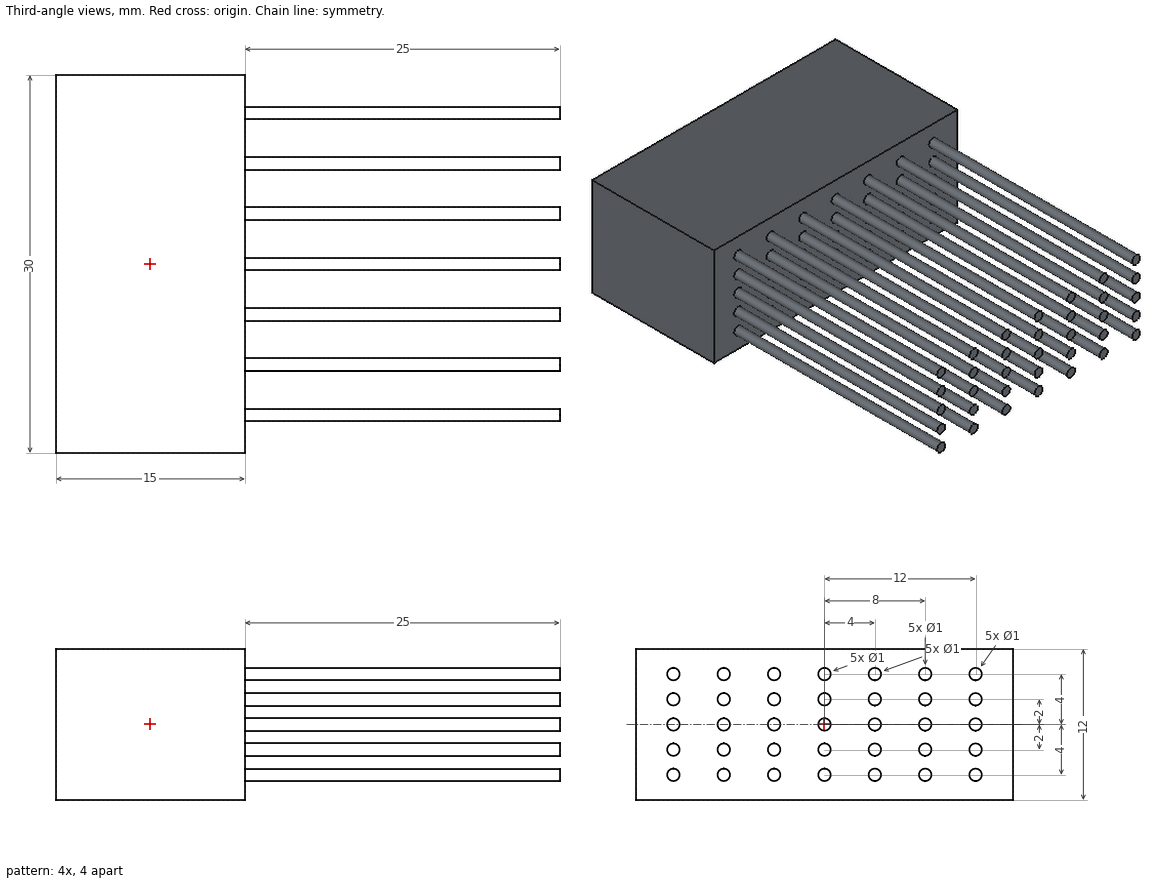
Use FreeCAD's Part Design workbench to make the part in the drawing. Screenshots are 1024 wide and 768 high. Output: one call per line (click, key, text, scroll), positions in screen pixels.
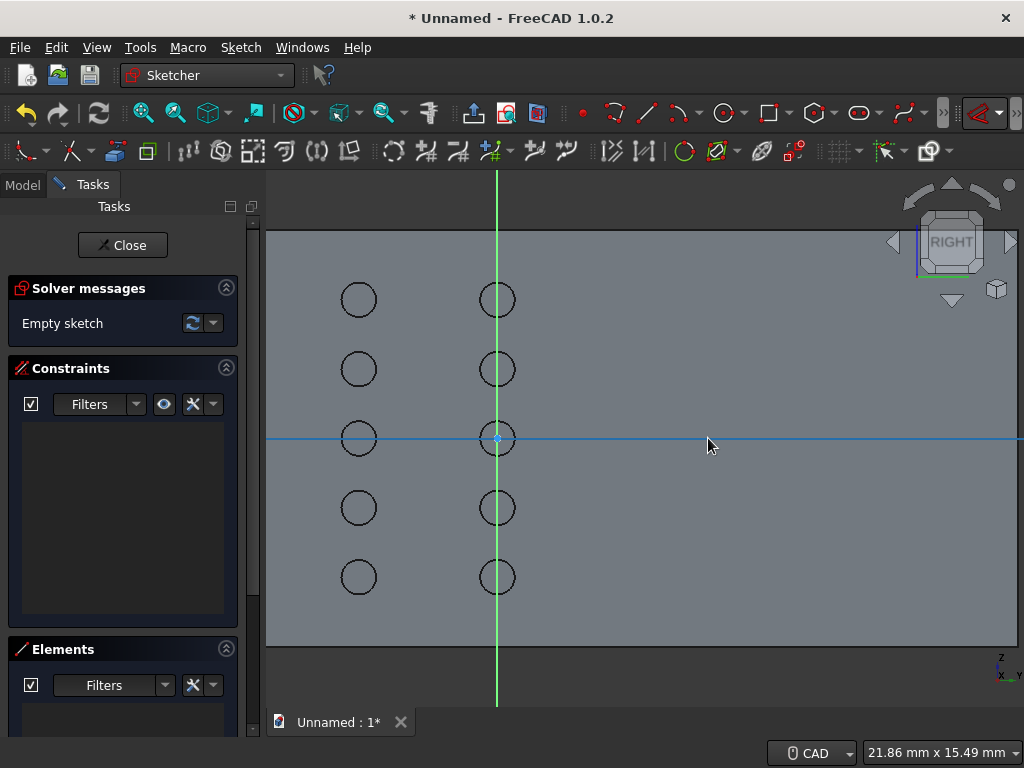
key(g)
key(c)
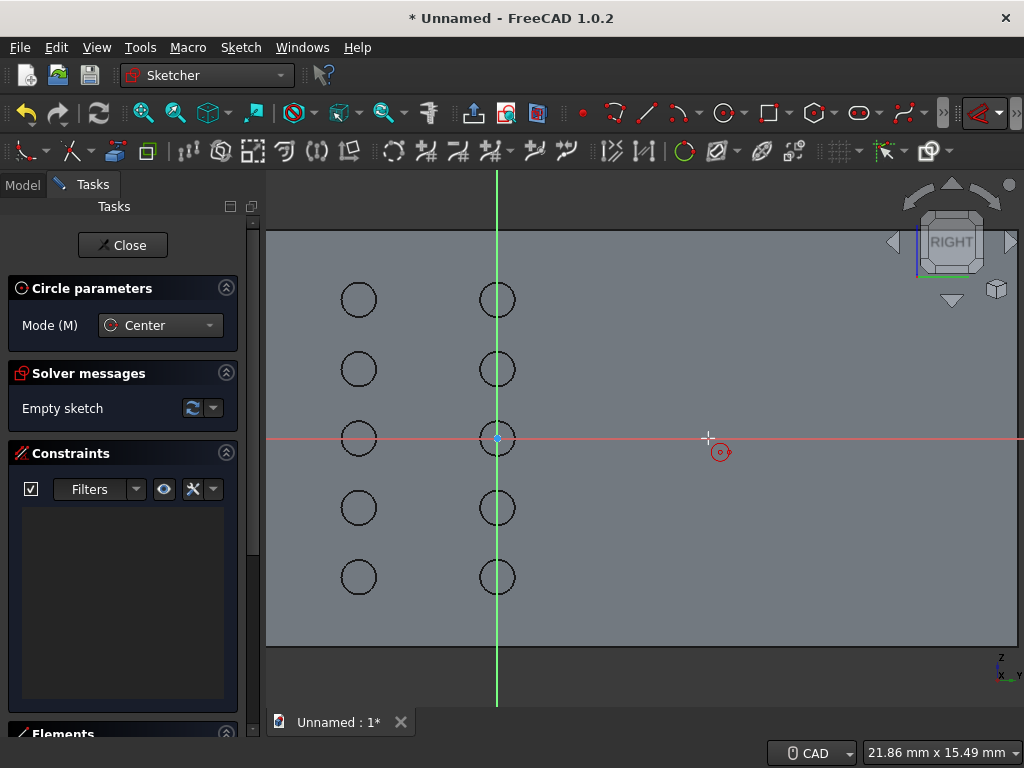
scroll(636, 300, up, 2)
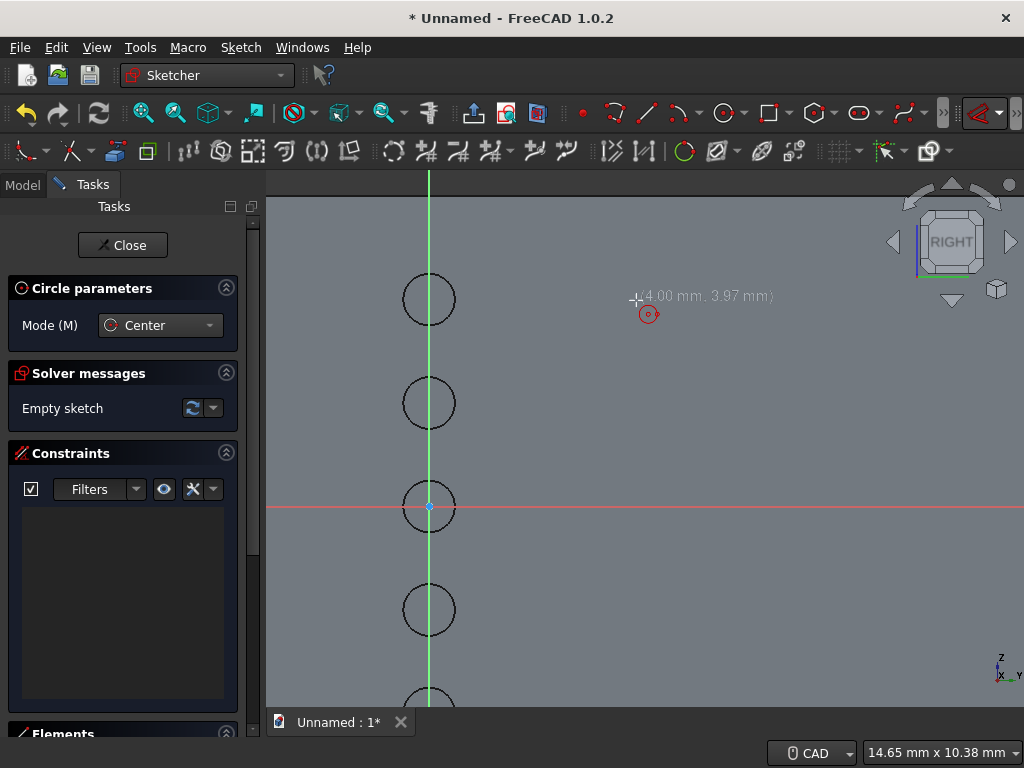
click(636, 300)
move(654, 281)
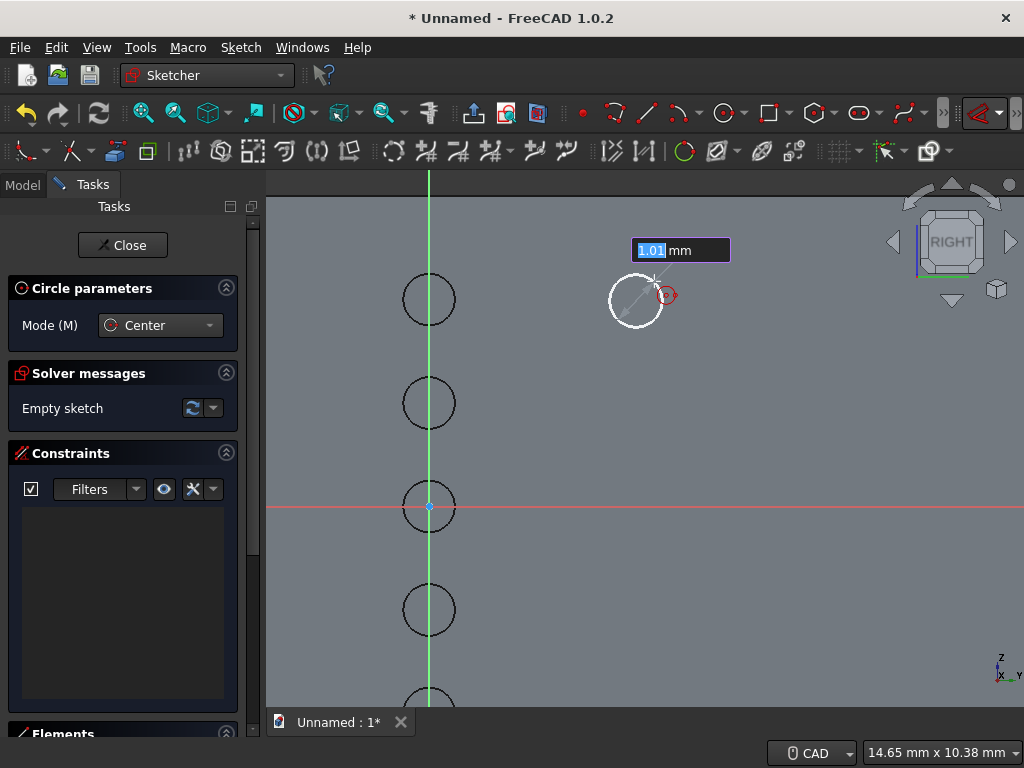
text(1)
key(Return)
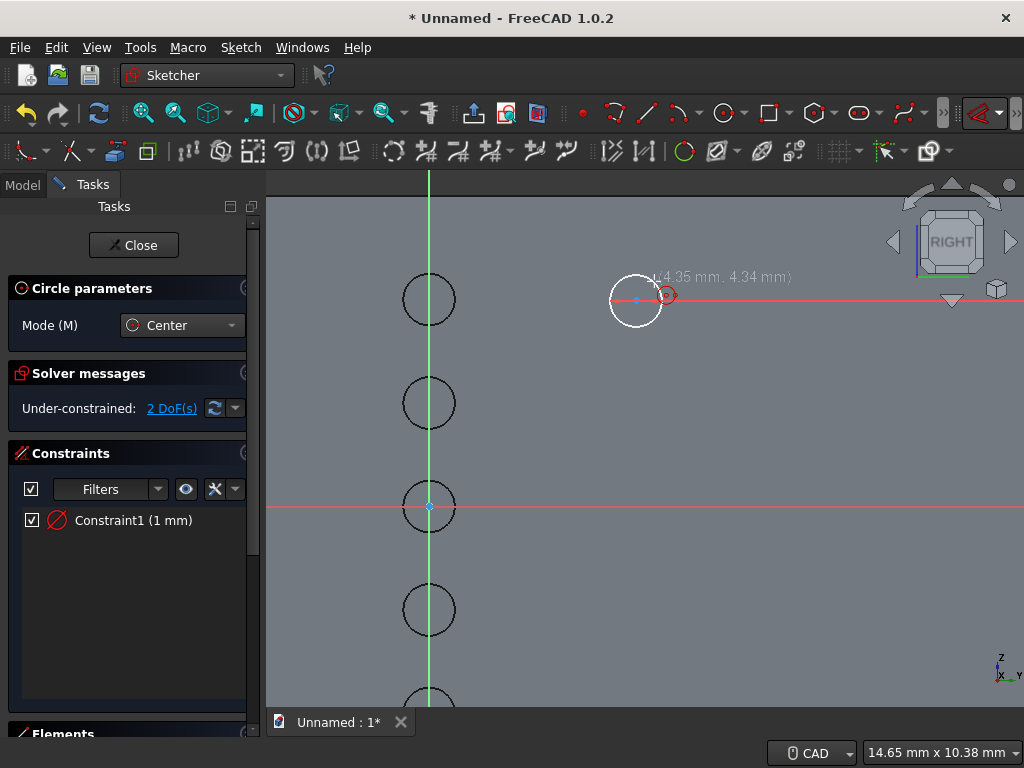
click(636, 403)
move(654, 385)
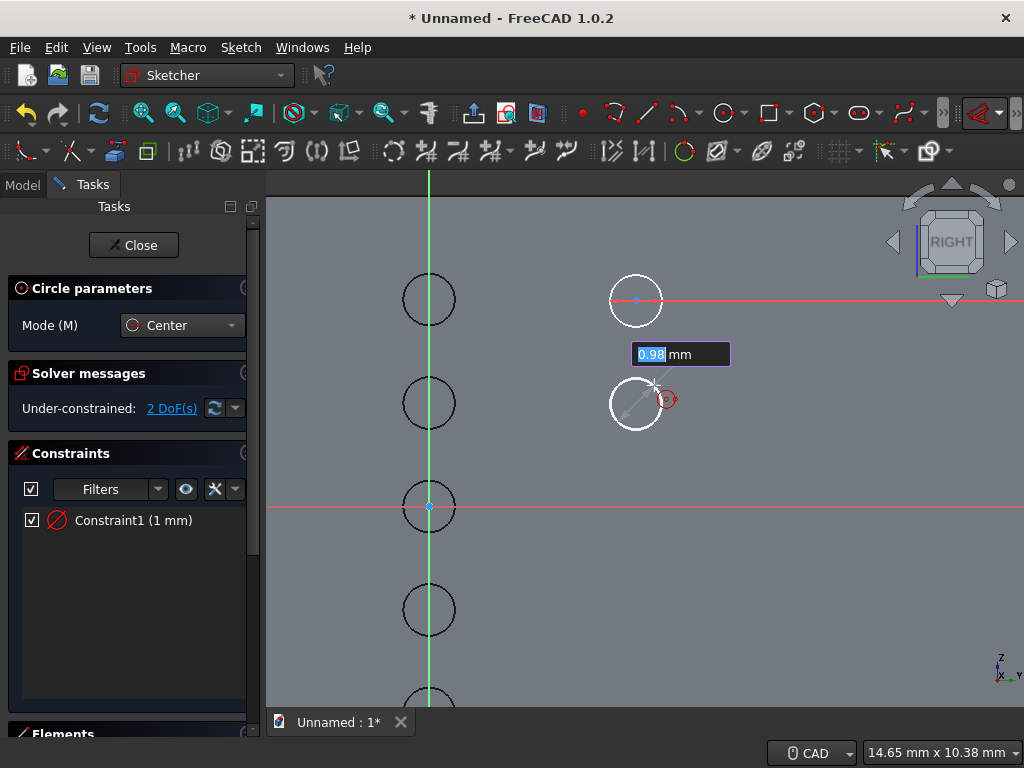
text(1)
key(Return)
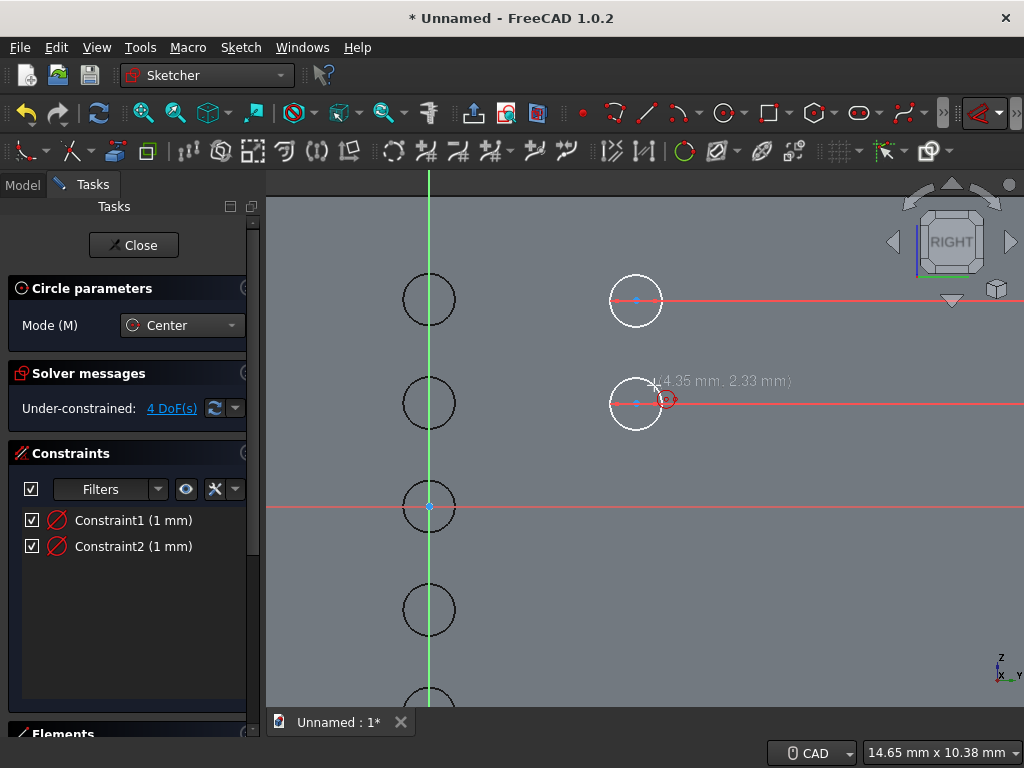
click(636, 506)
move(654, 488)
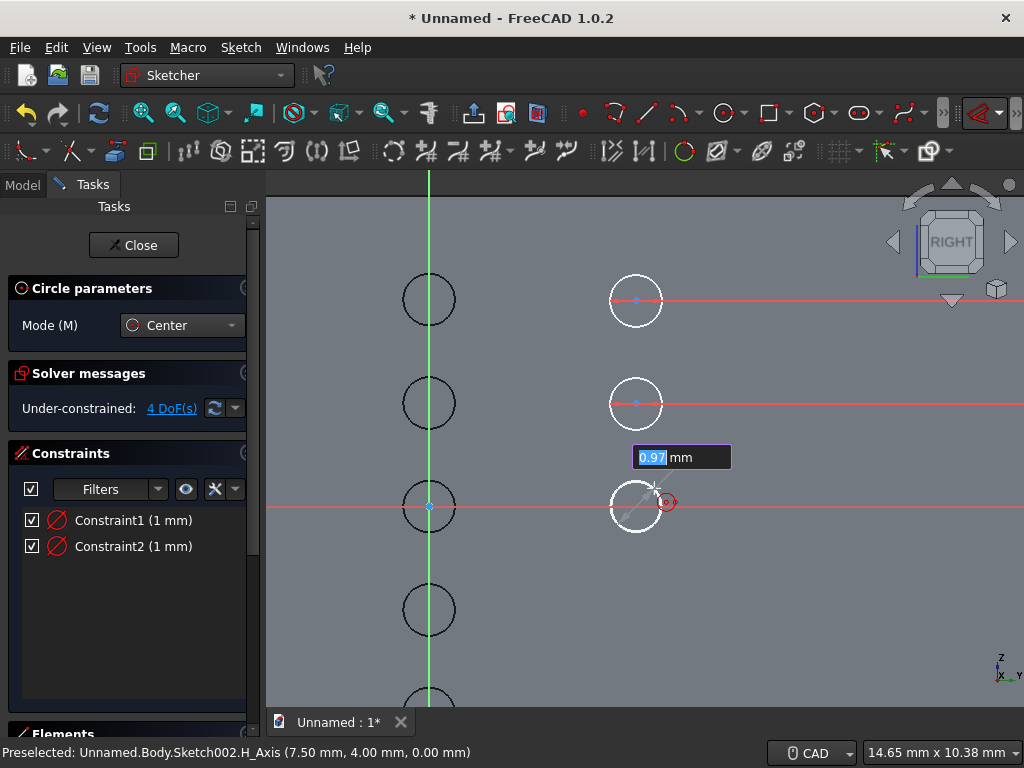
text(1)
key(Return)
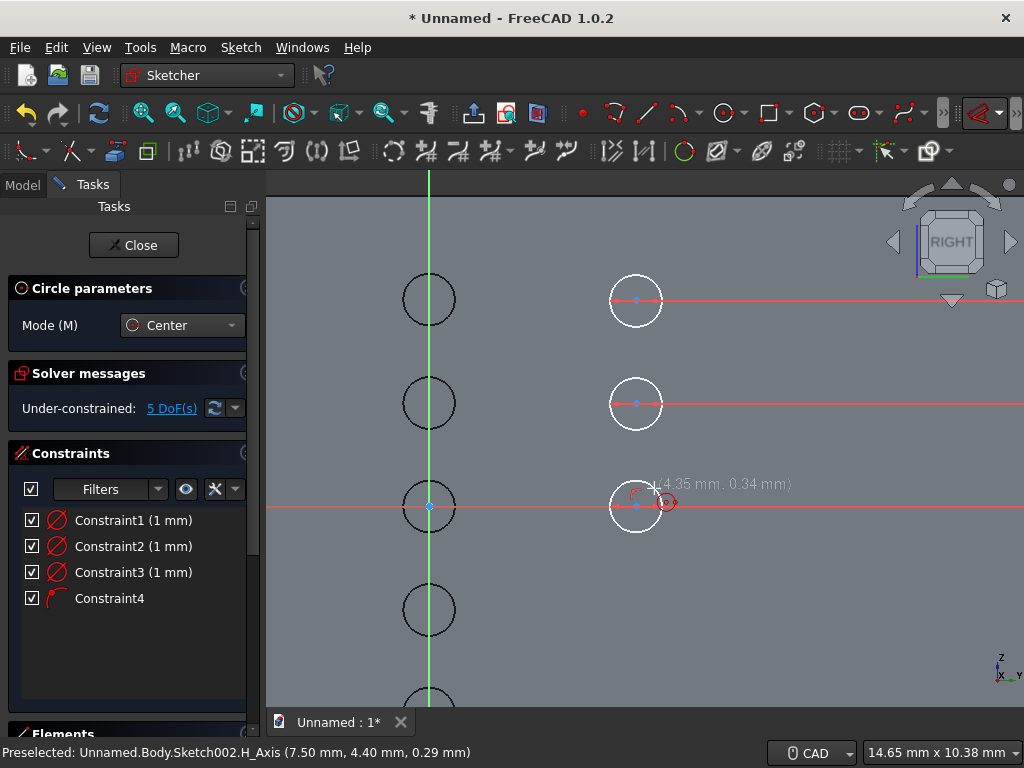
click(636, 610)
move(654, 592)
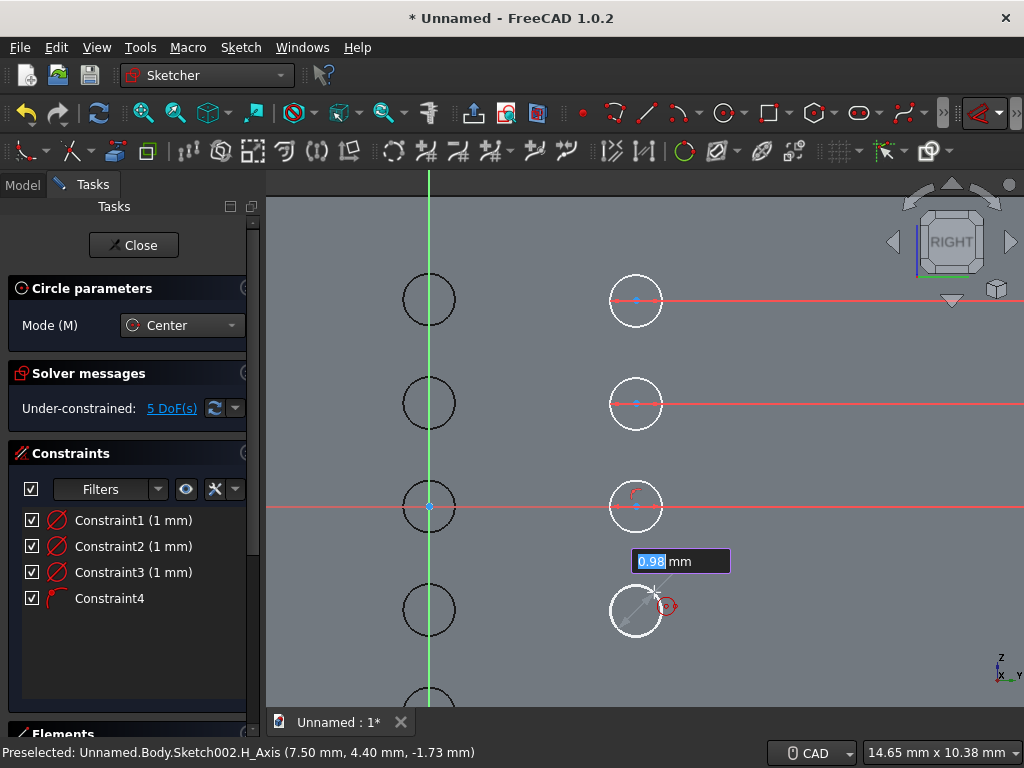
text(1)
key(Return)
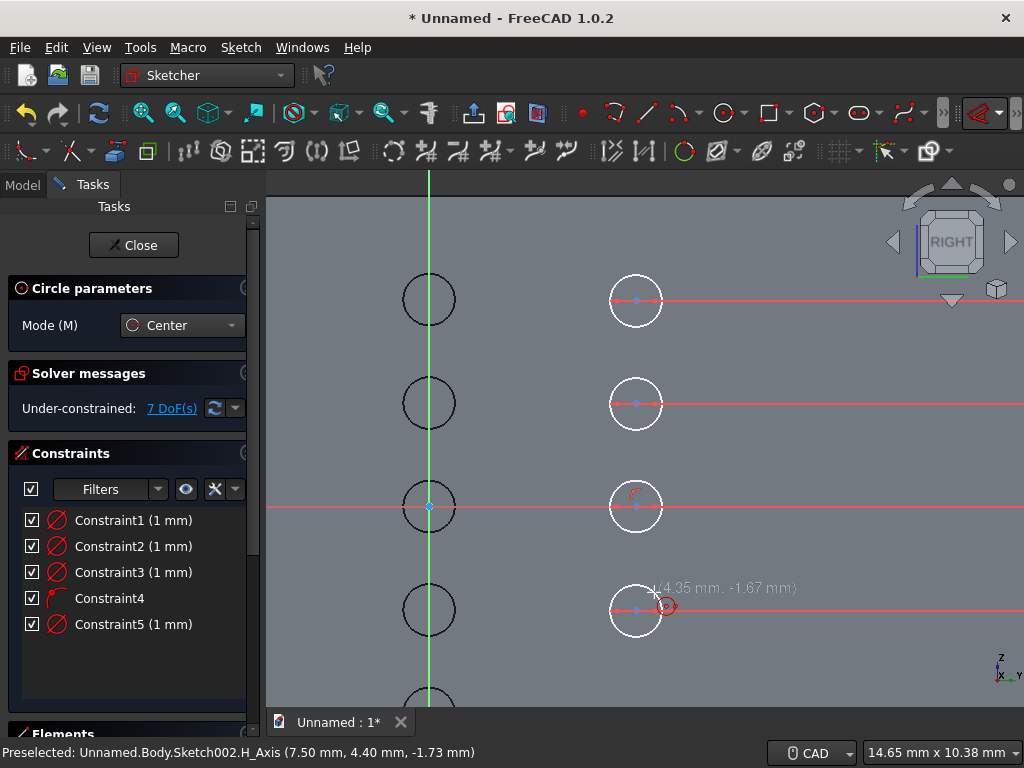
scroll(640, 300, down, 2)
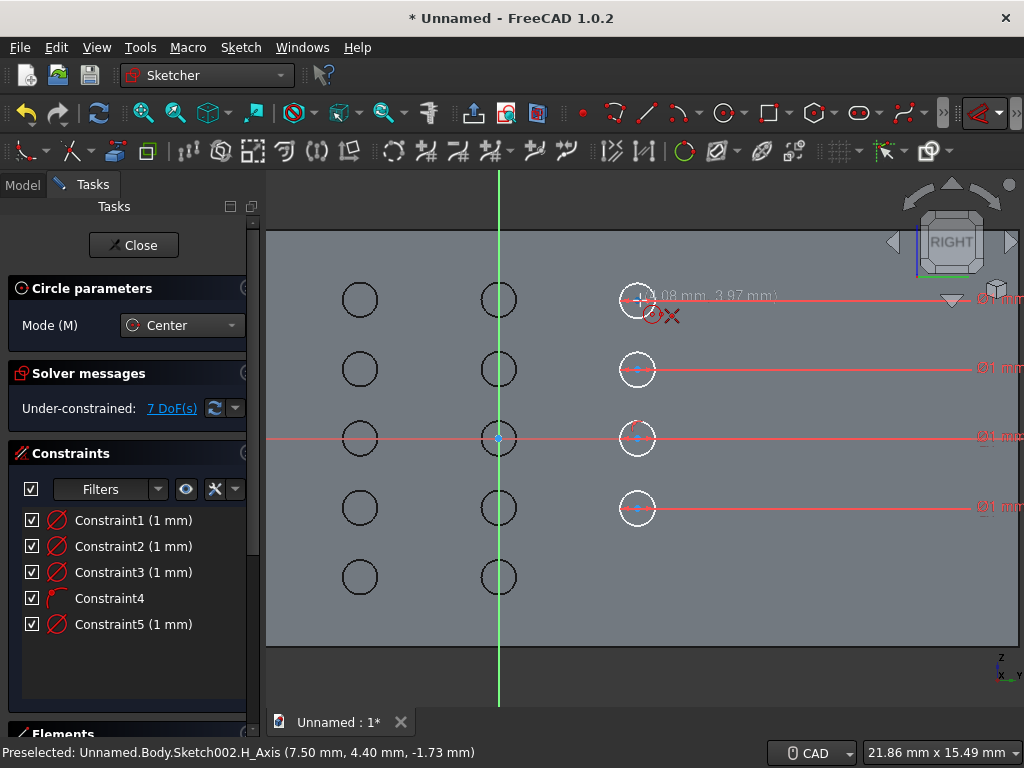
scroll(637, 577, up, 2)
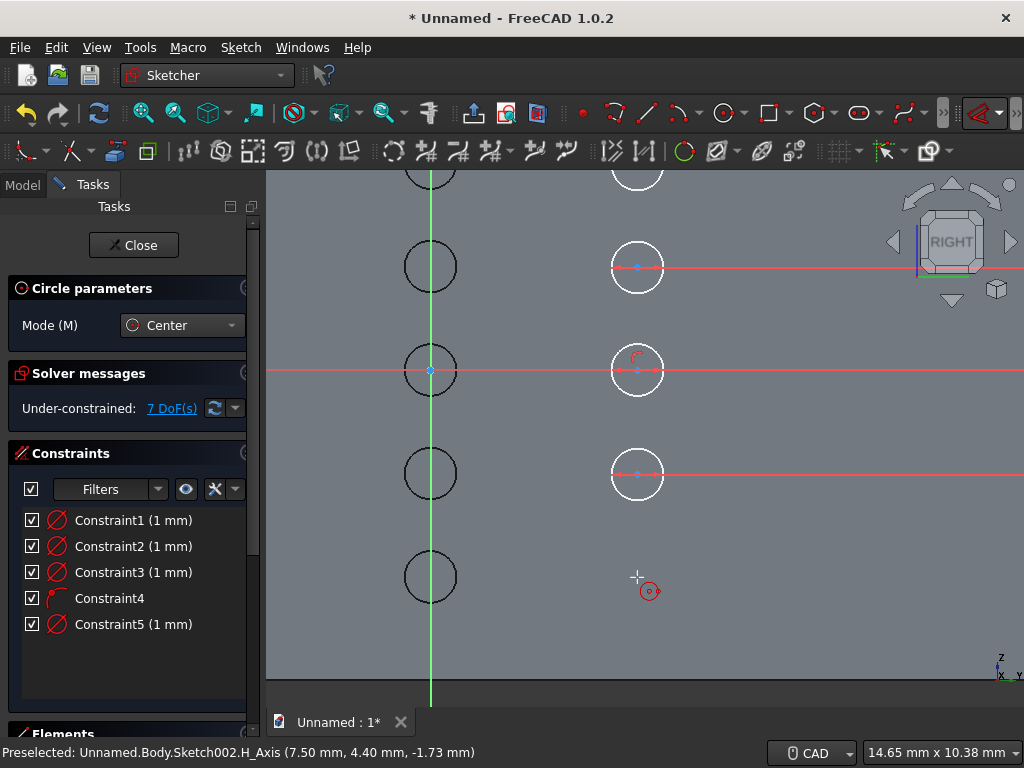
click(637, 577)
move(656, 559)